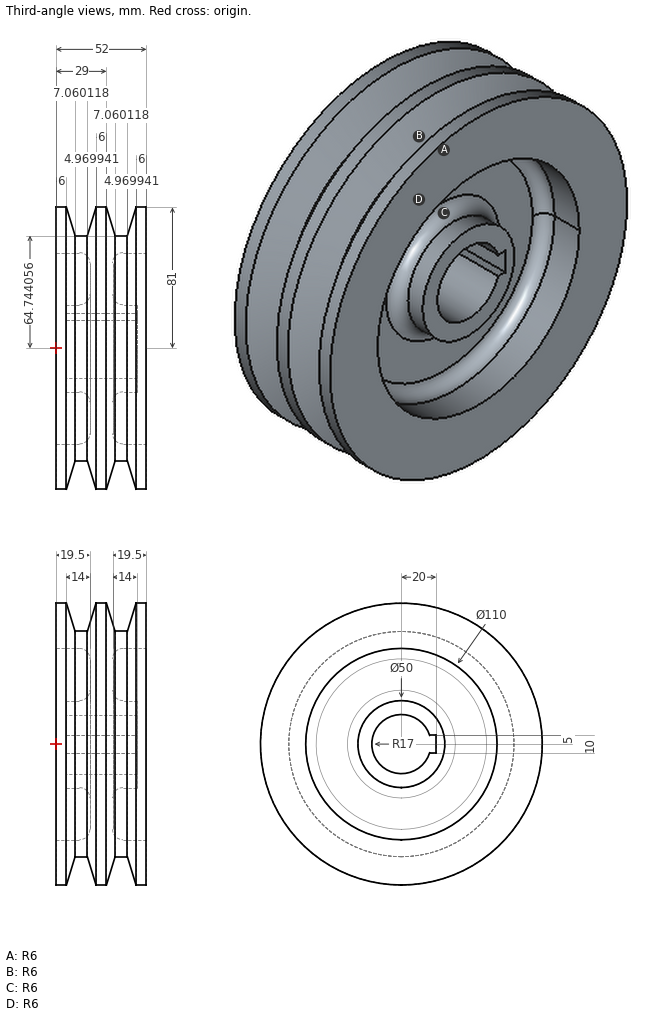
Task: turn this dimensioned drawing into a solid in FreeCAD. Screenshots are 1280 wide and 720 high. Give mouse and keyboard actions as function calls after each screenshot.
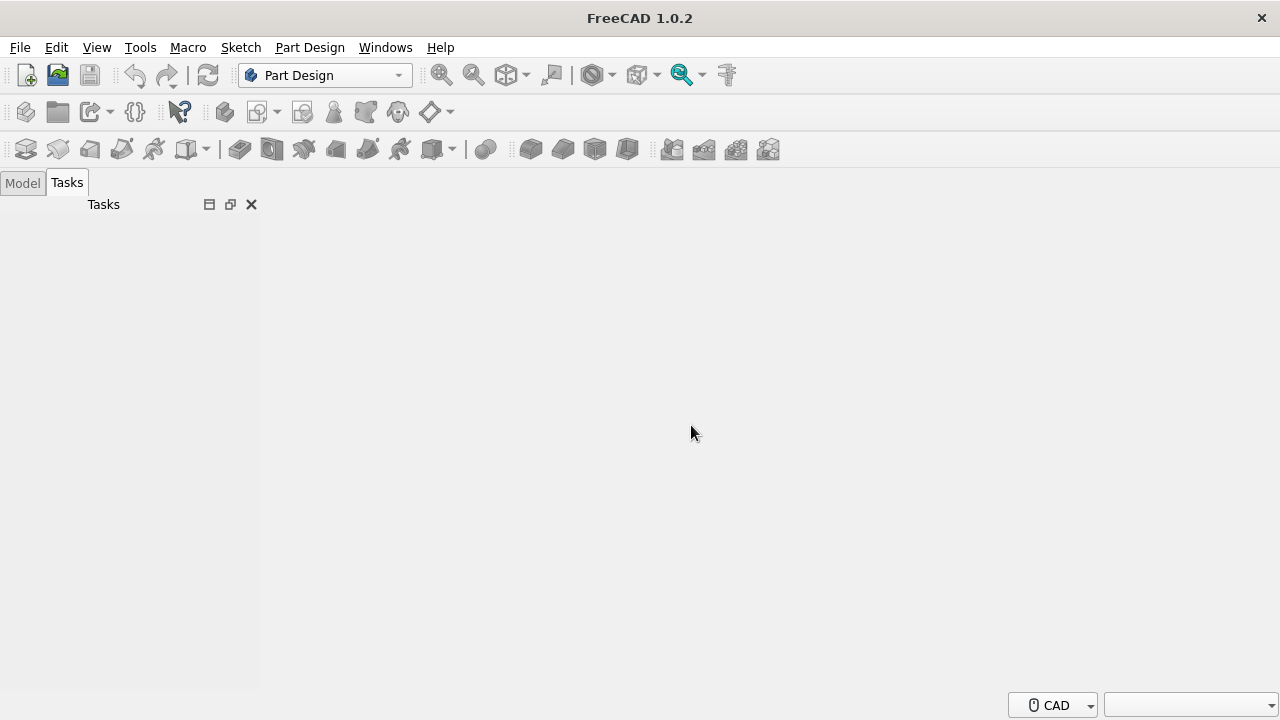
key(ctrl+n)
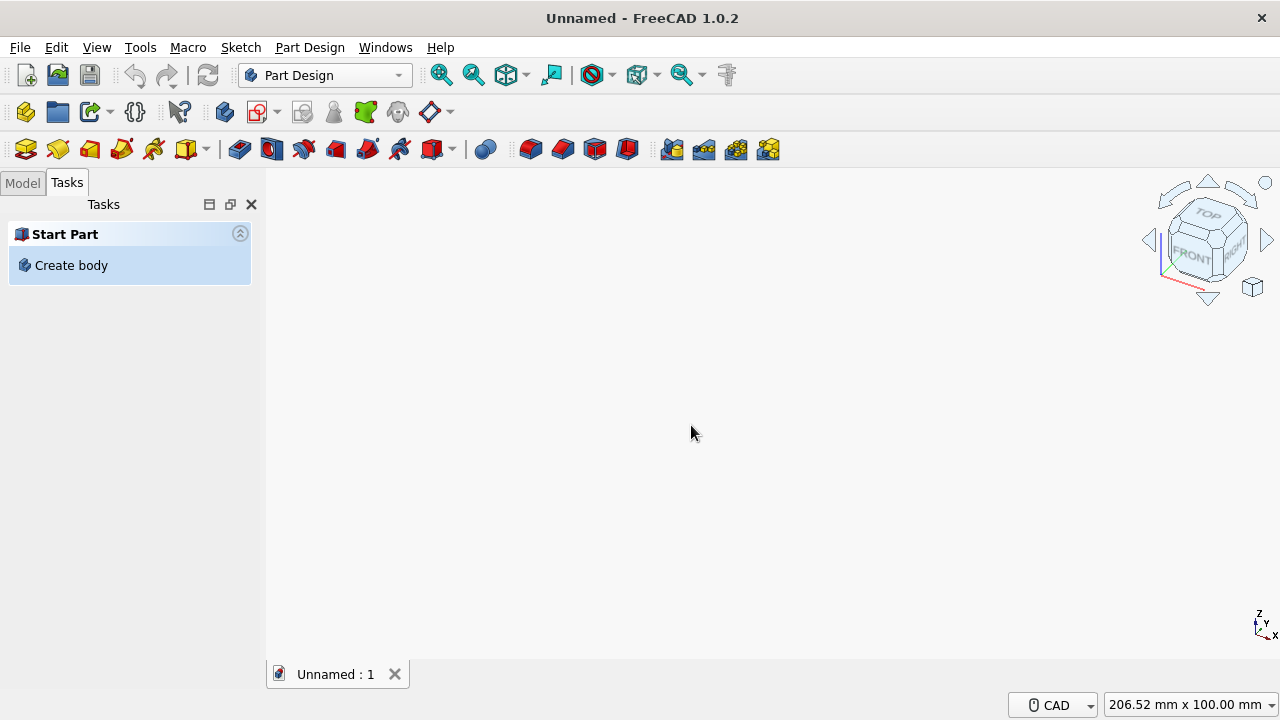
click(258, 112)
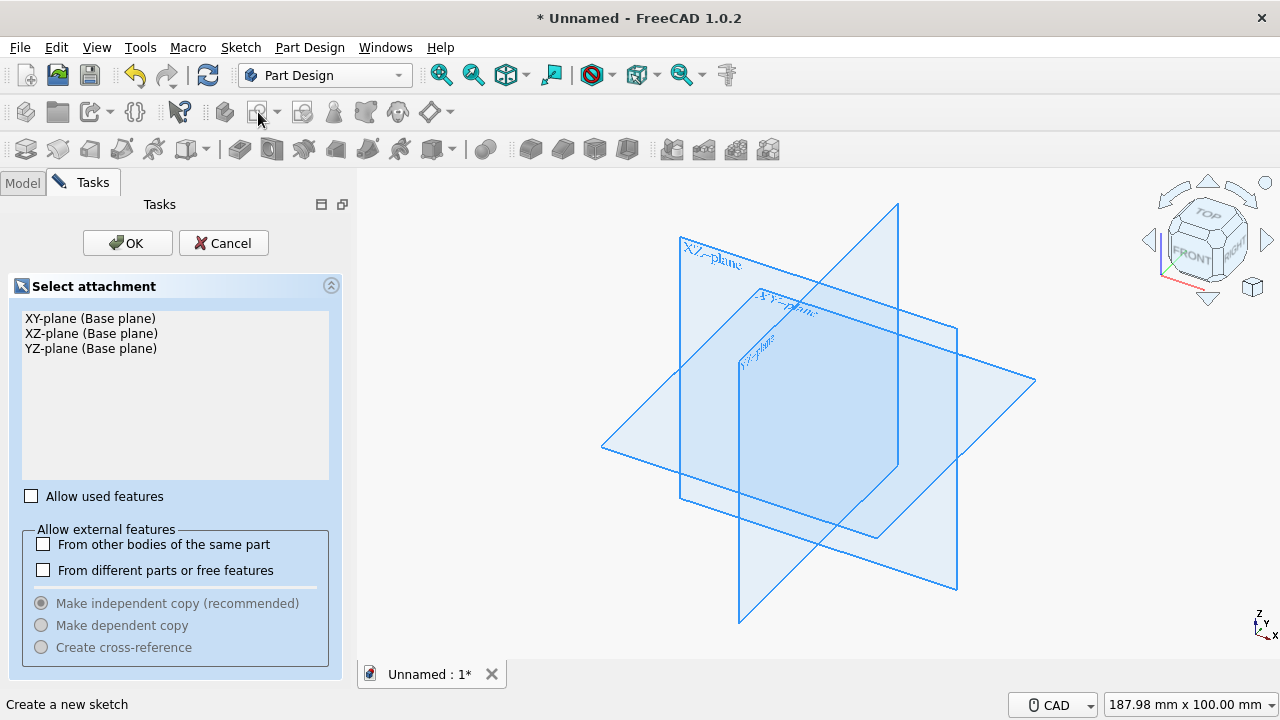
click(82, 318)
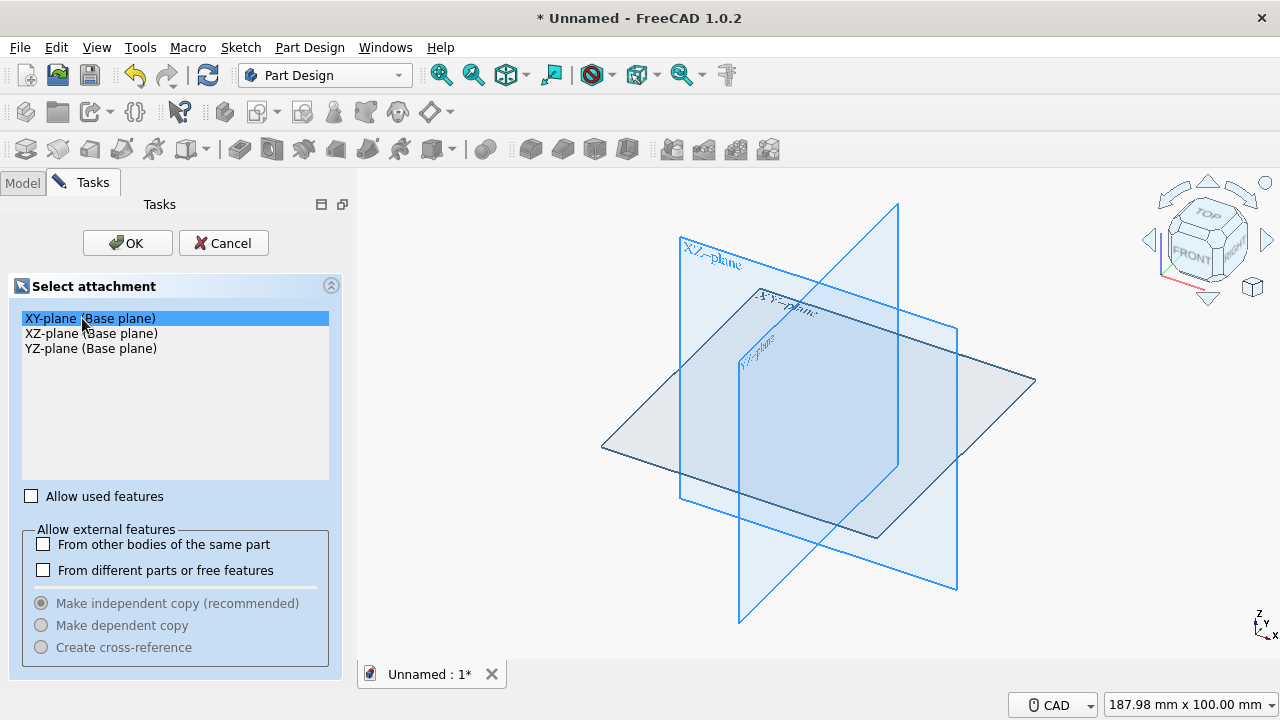
click(128, 243)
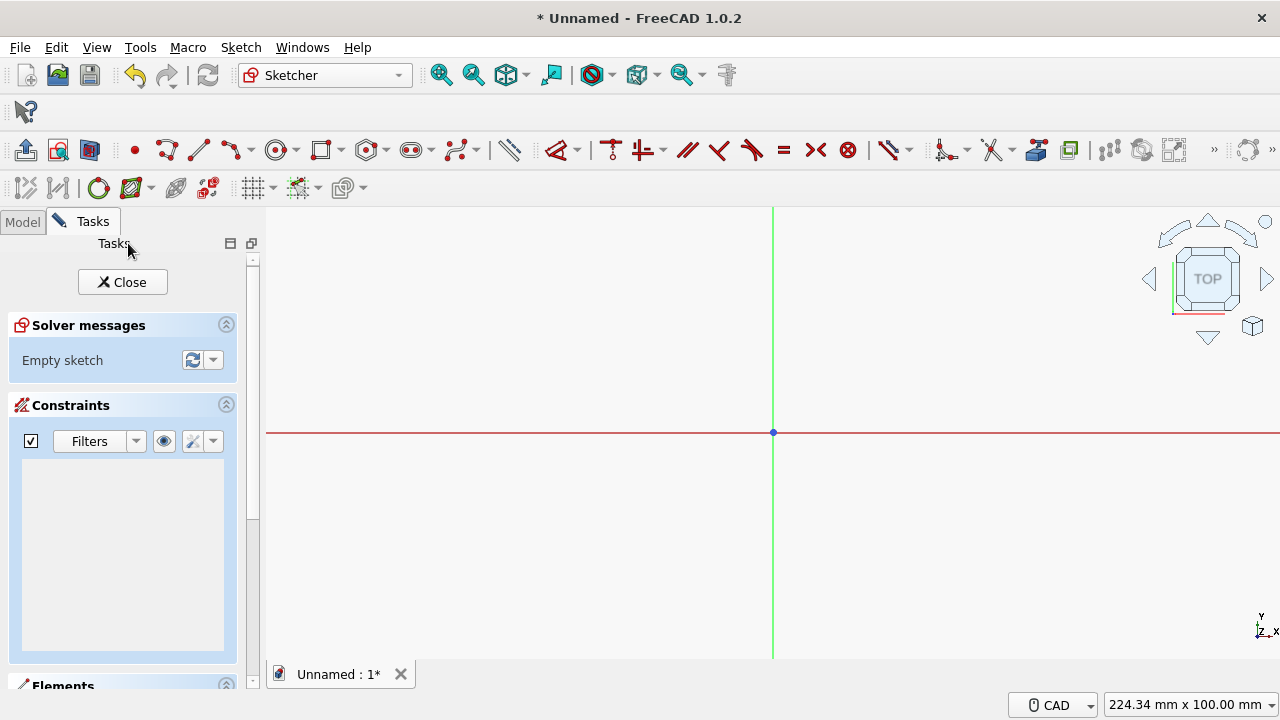
scroll(478, 631, down, 3)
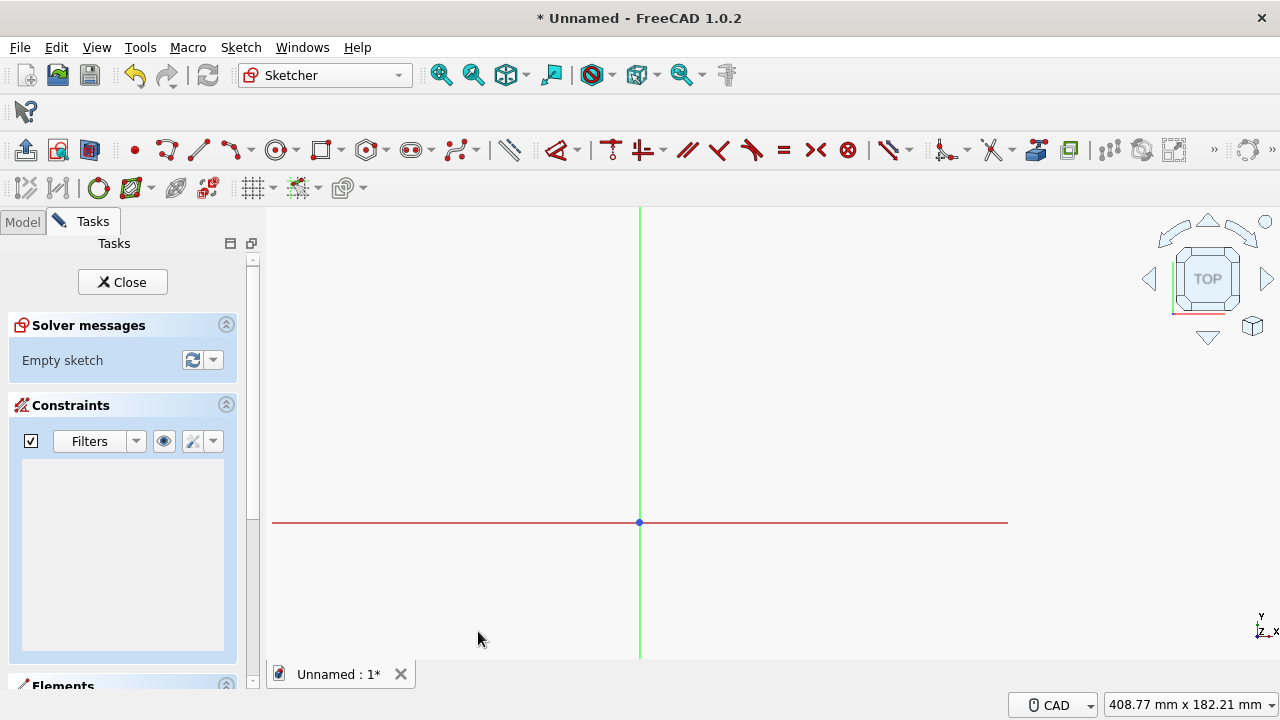
scroll(704, 401, up, 2)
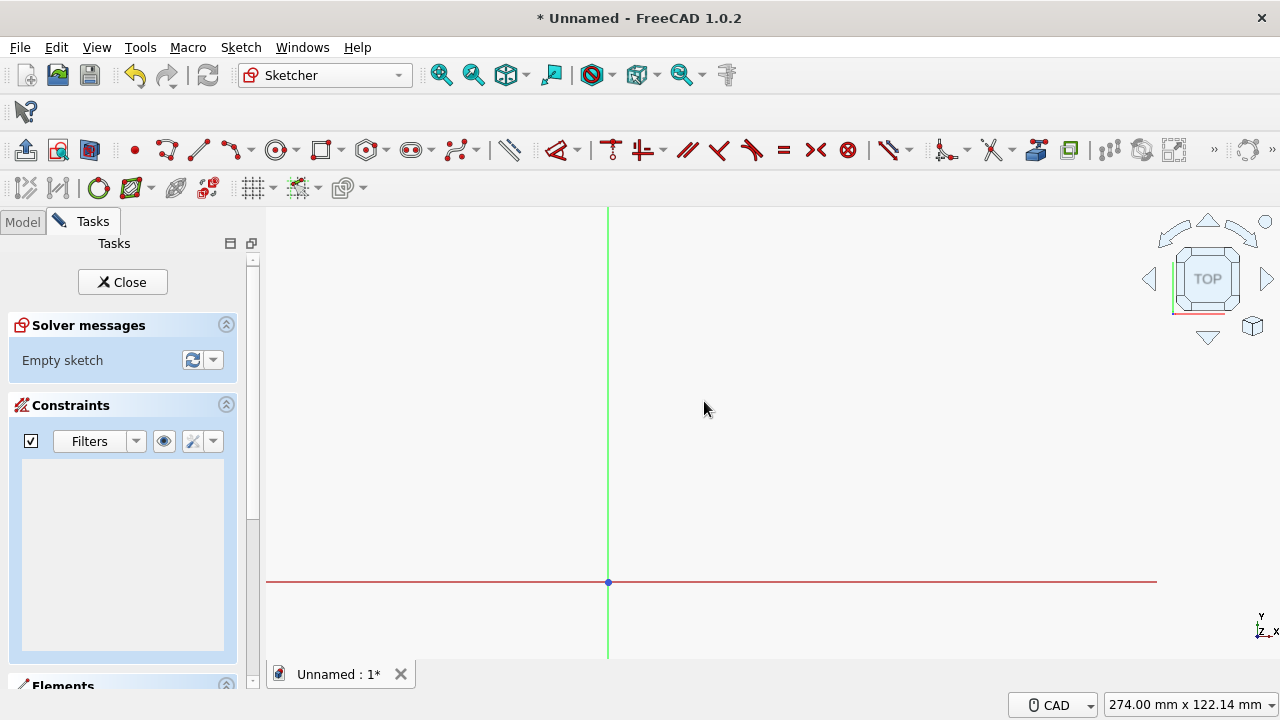
key(g)
key(m)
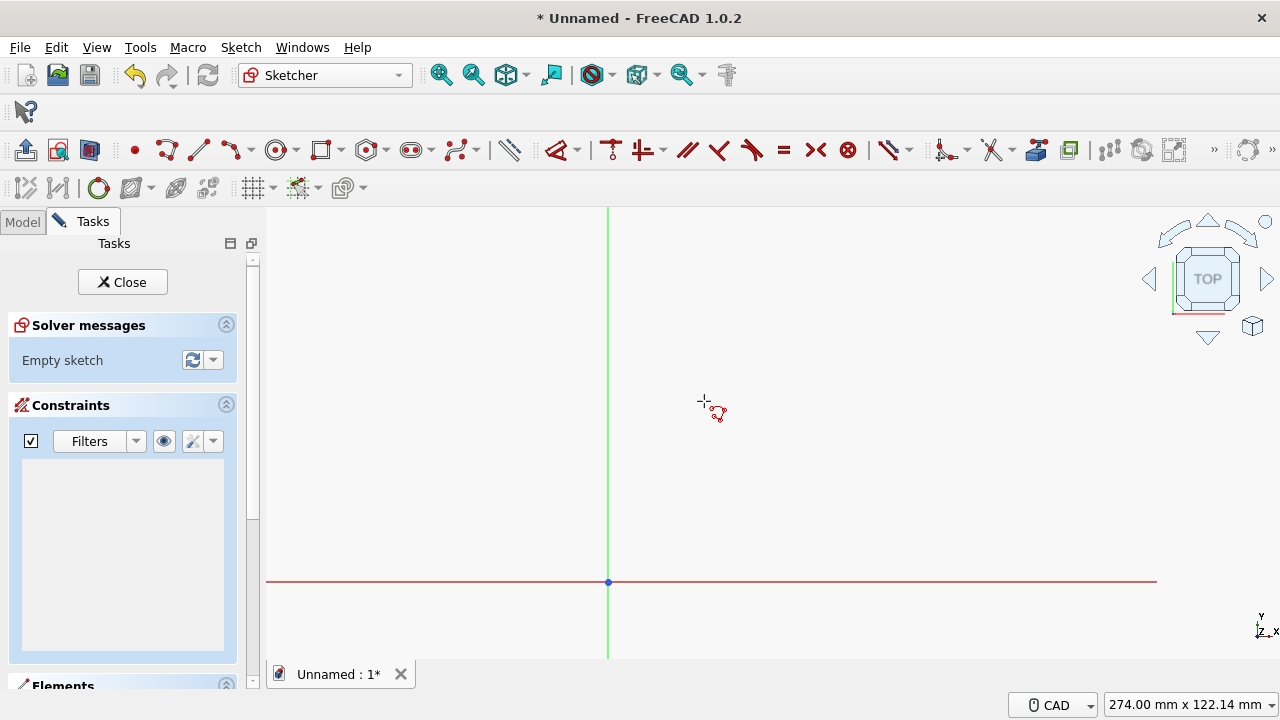
click(608, 582)
click(801, 573)
click(801, 283)
click(779, 283)
click(760, 343)
click(734, 343)
click(716, 283)
click(693, 283)
click(675, 343)
click(649, 343)
click(631, 283)
click(617, 283)
click(608, 582)
key(Escape)
key(Escape)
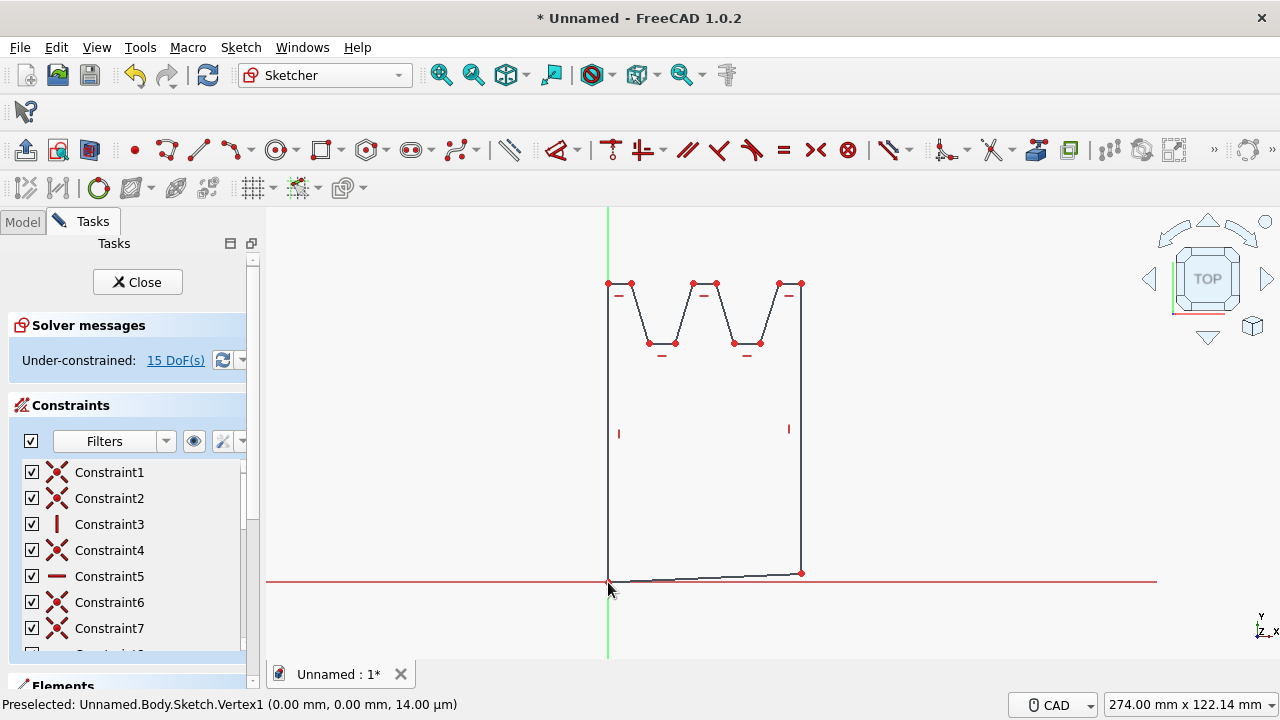
click(666, 580)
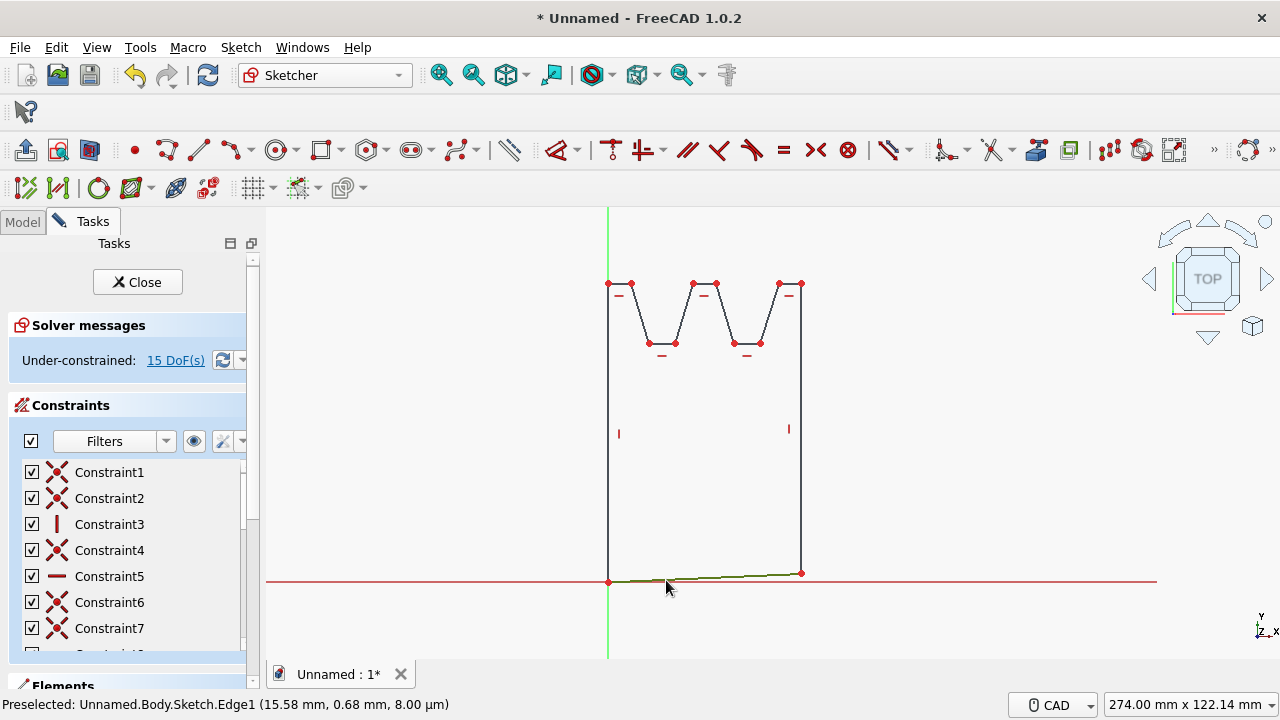
key(h)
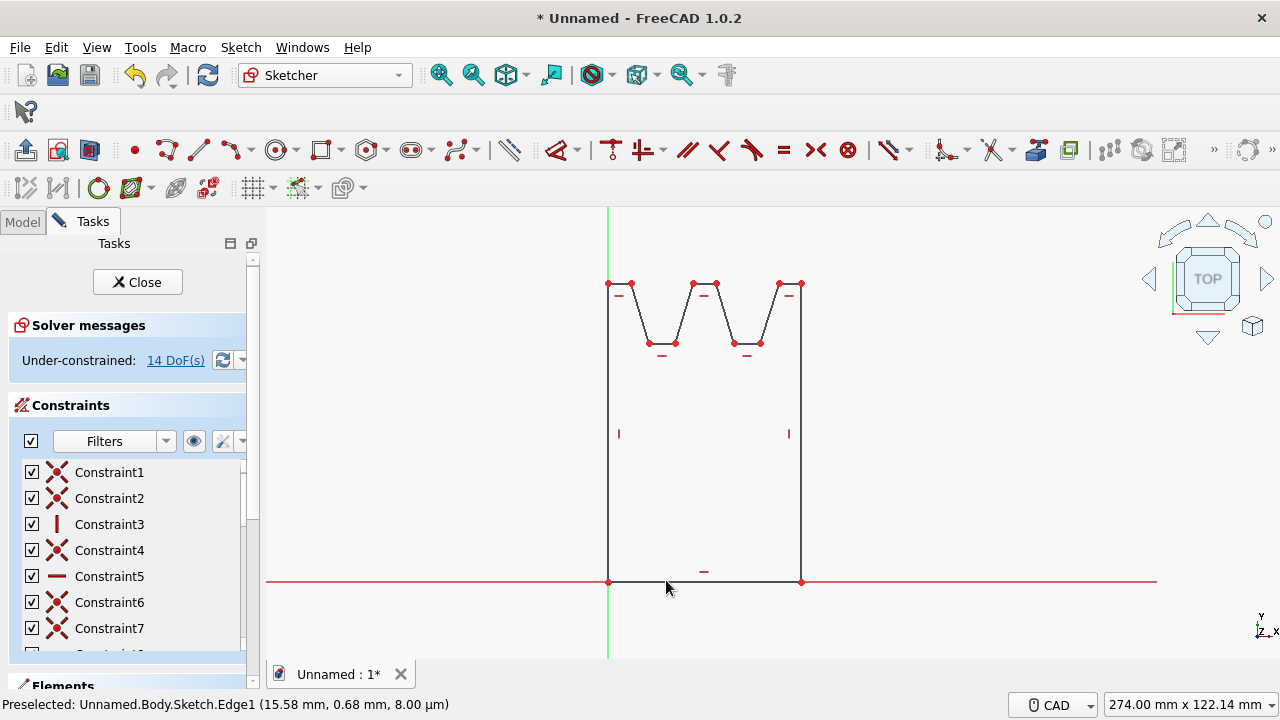
key(d)